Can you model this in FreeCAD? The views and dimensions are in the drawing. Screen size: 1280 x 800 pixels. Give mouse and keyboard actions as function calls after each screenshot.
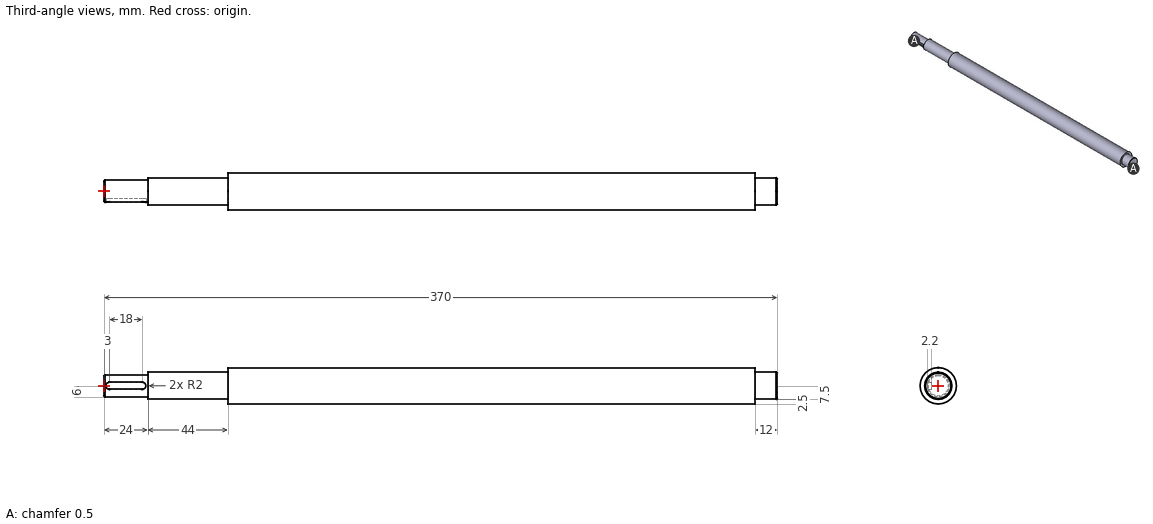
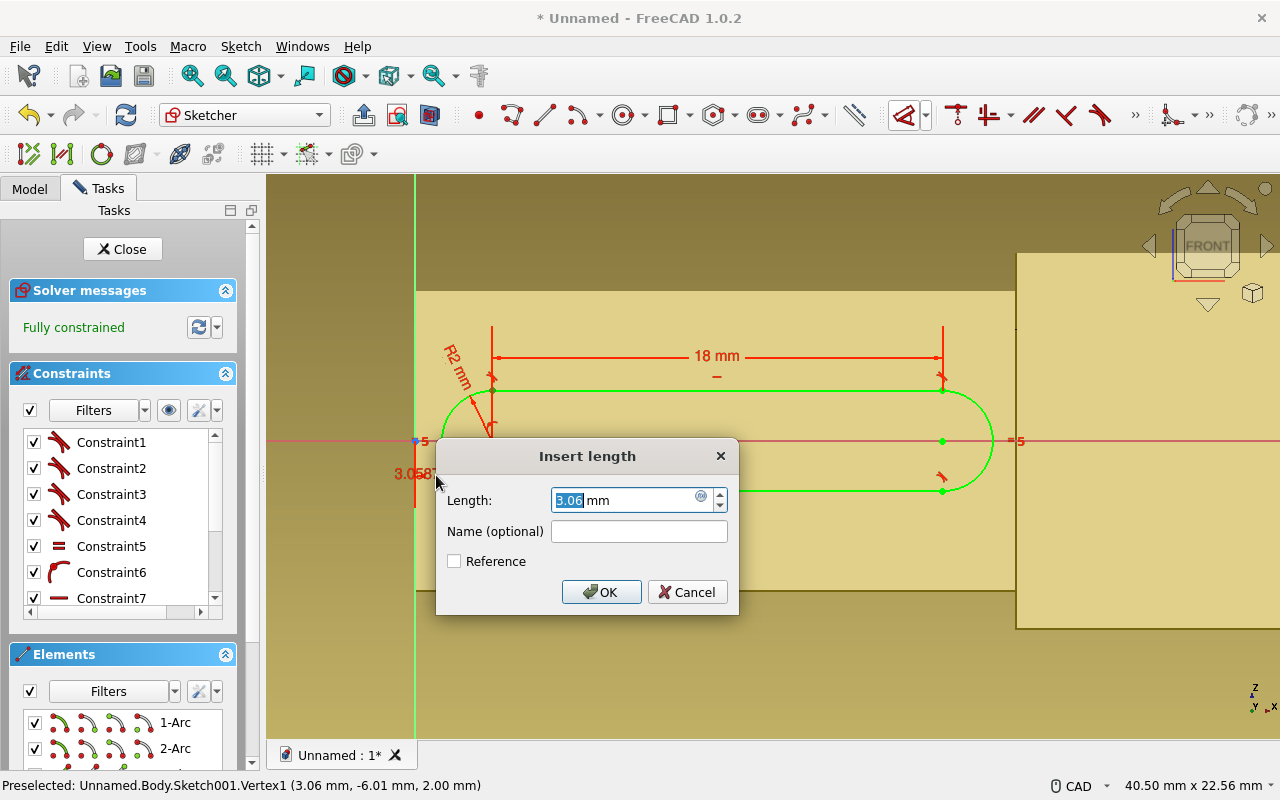
text(3)
key(Return)
key(Escape)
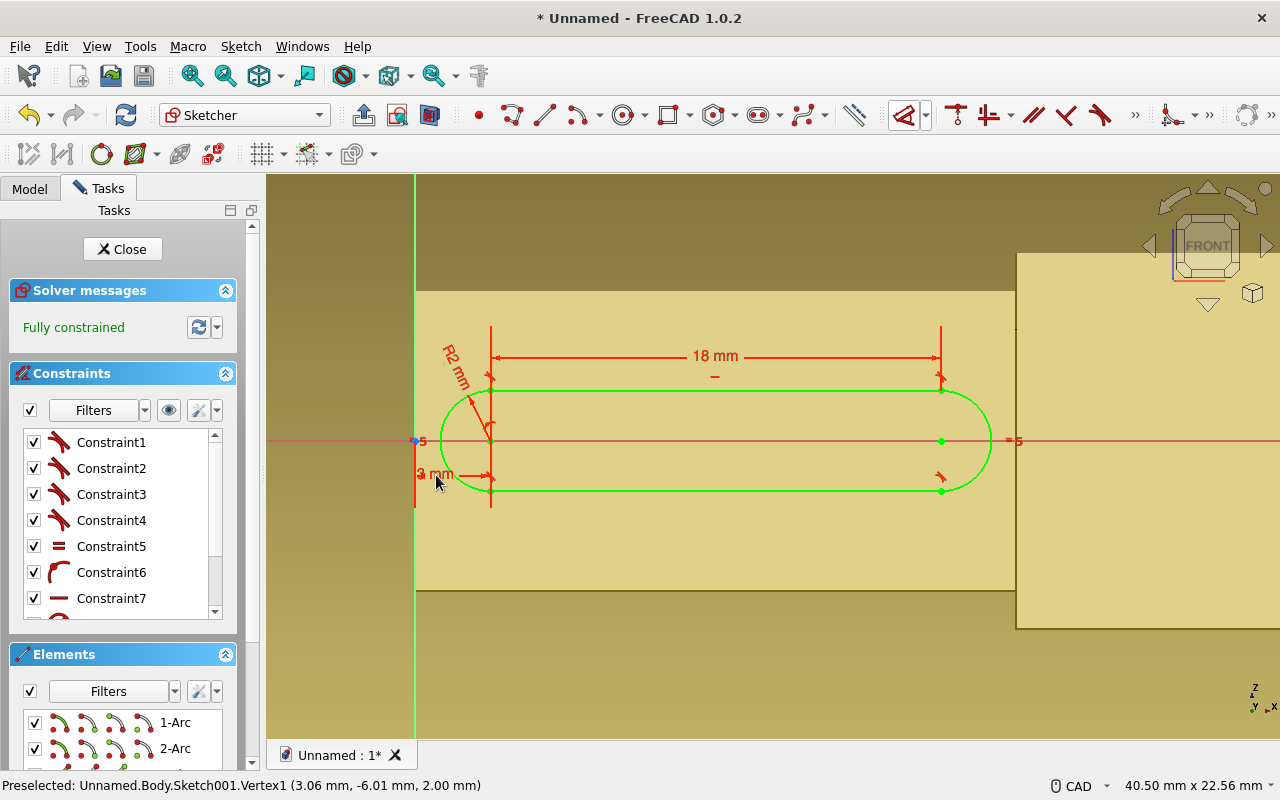
click(123, 249)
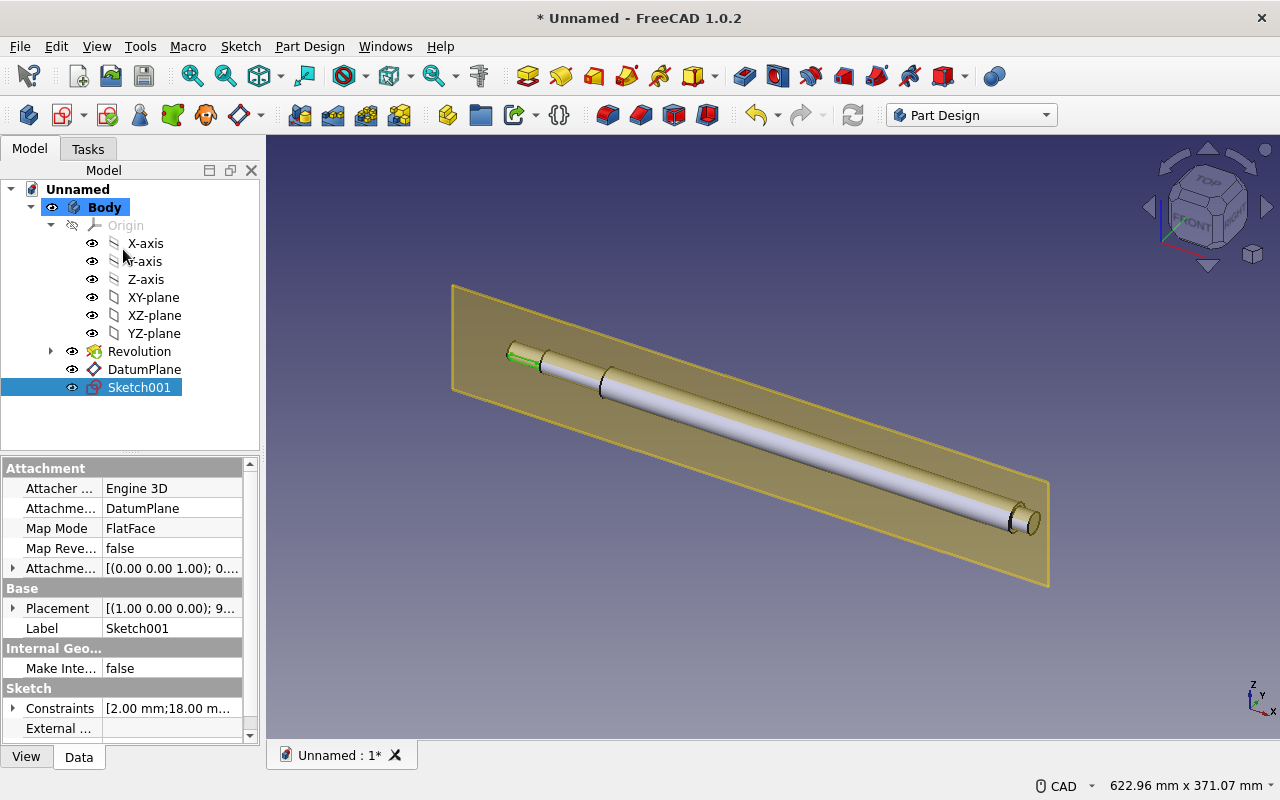
click(745, 76)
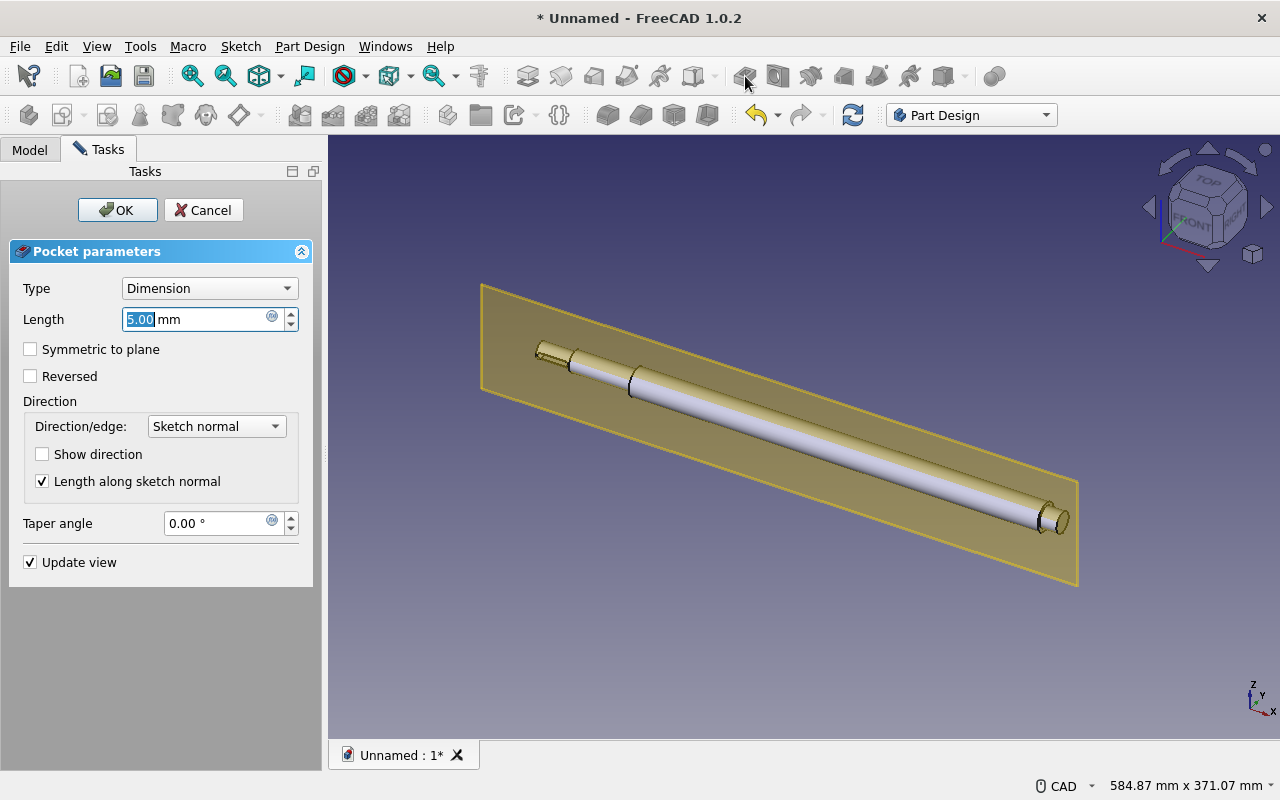
text(2.2)
key(Tab)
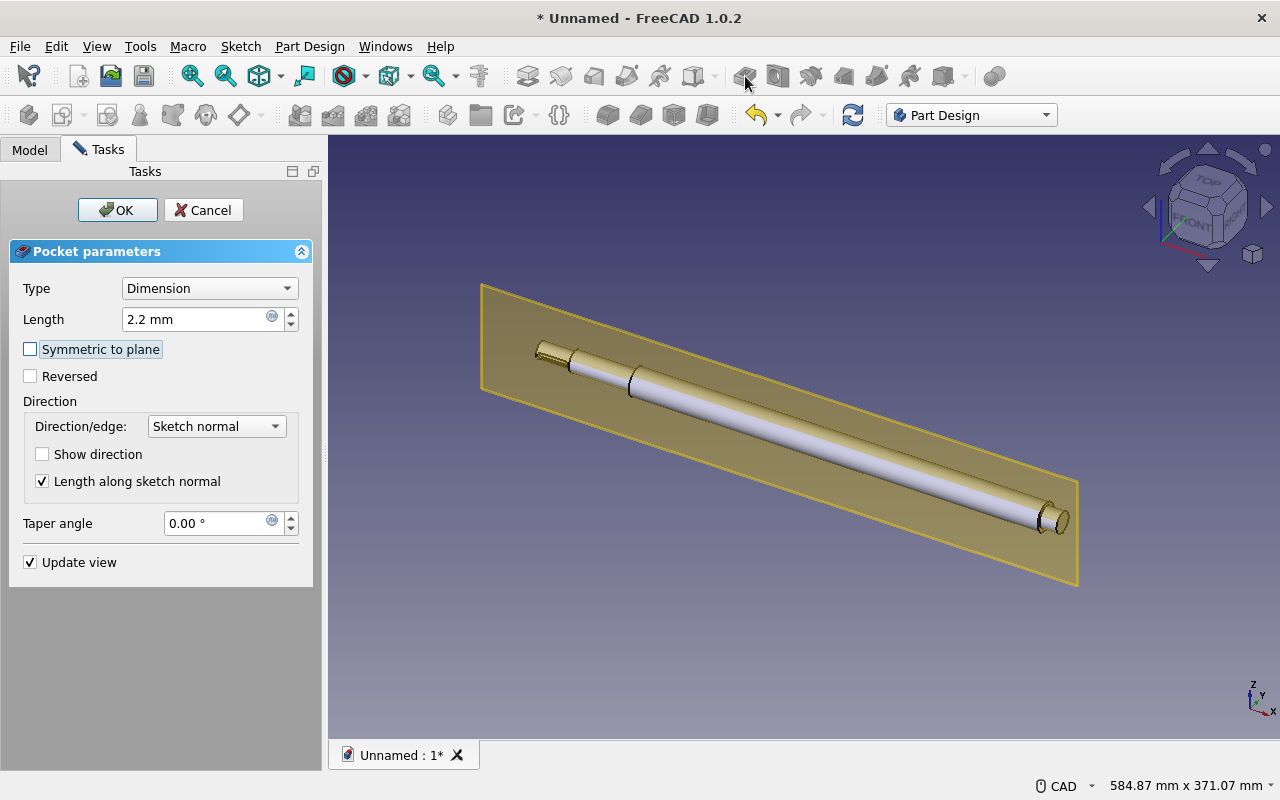
click(118, 210)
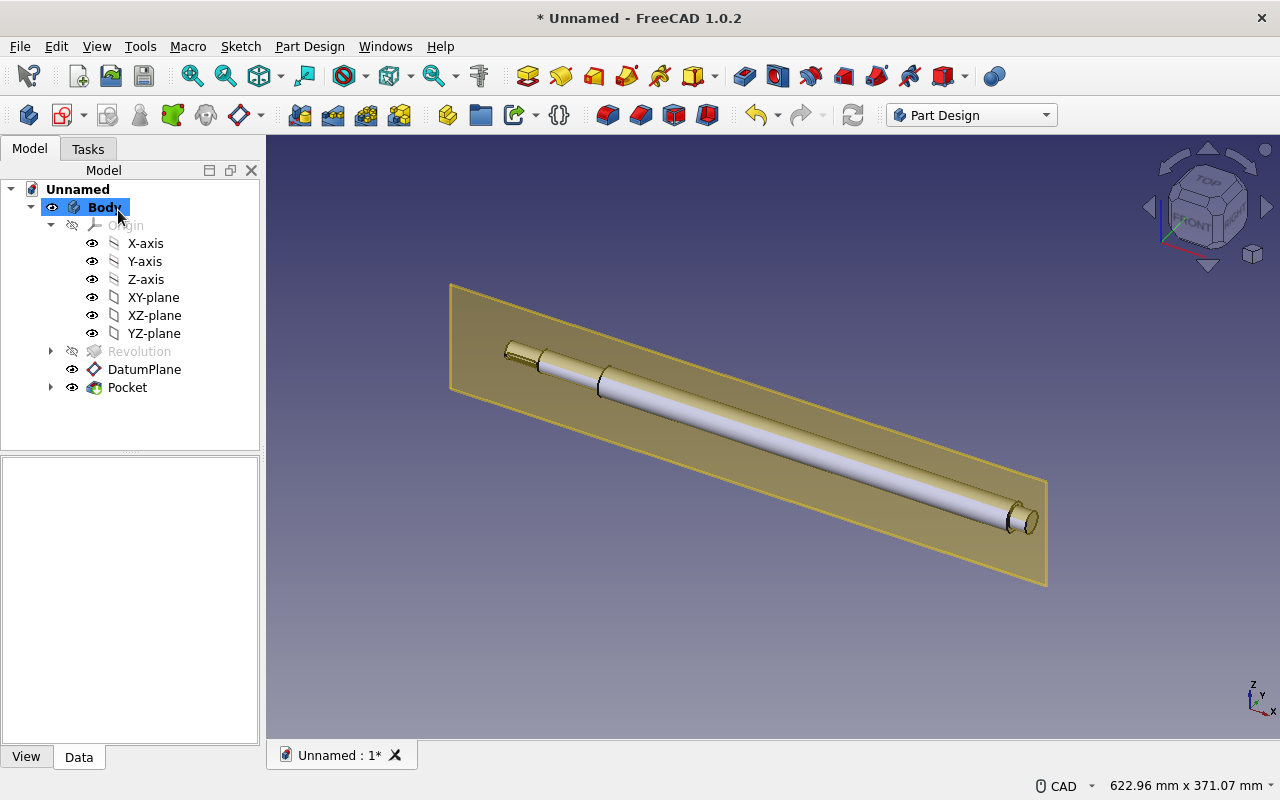
click(117, 369)
key(space)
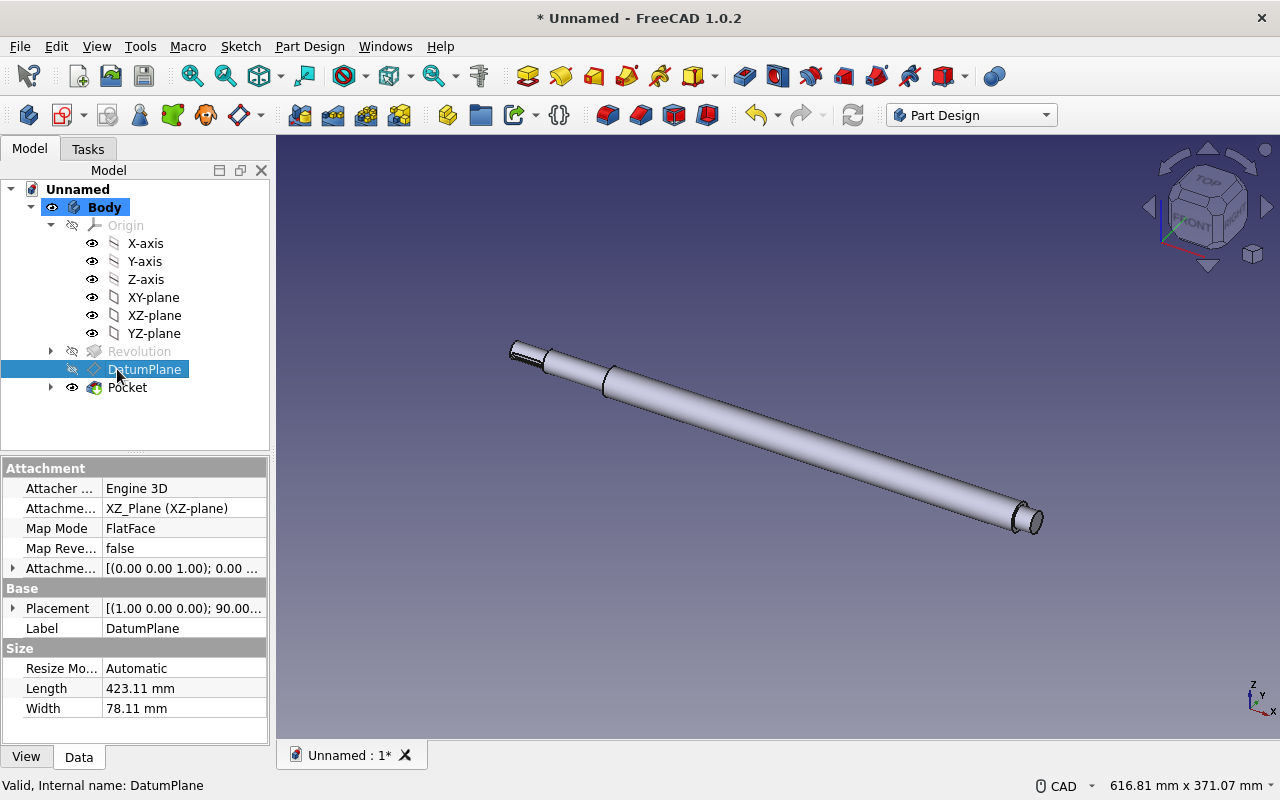
click(515, 341)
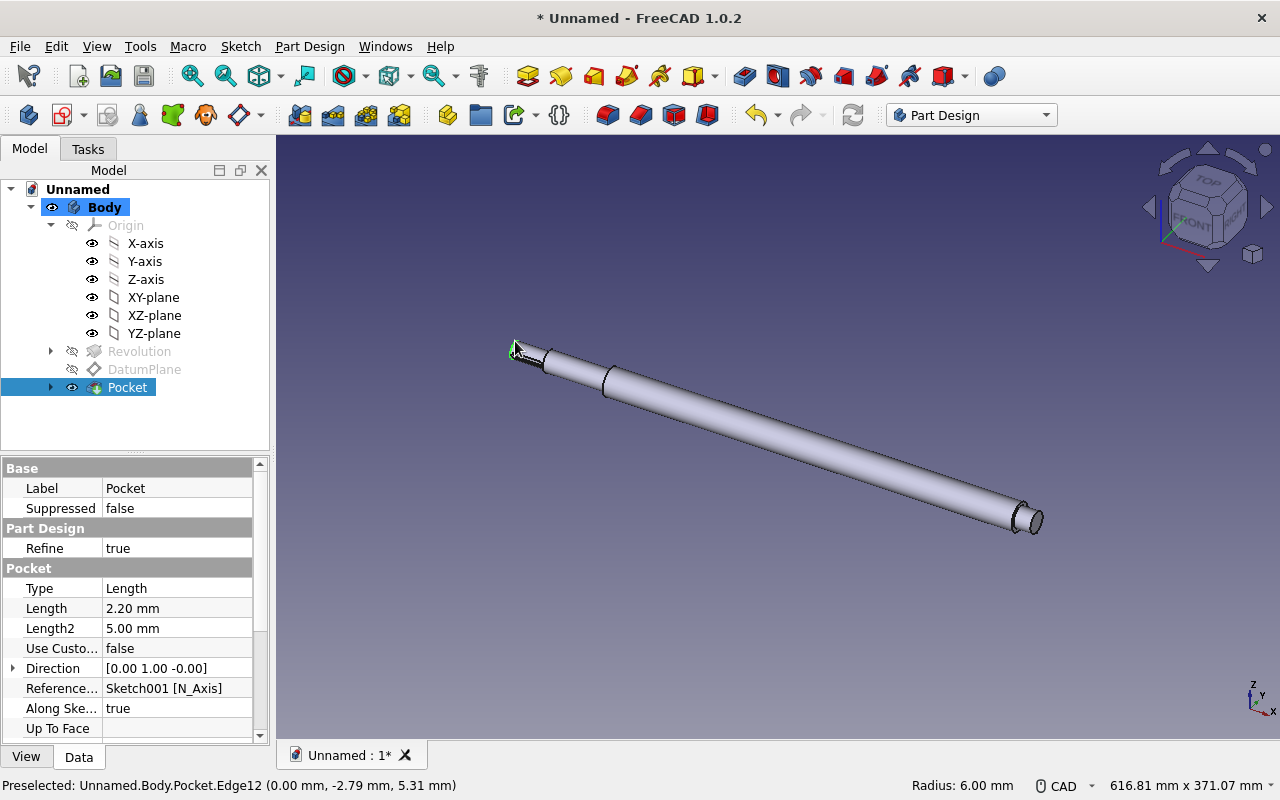
click(1037, 512, ctrl)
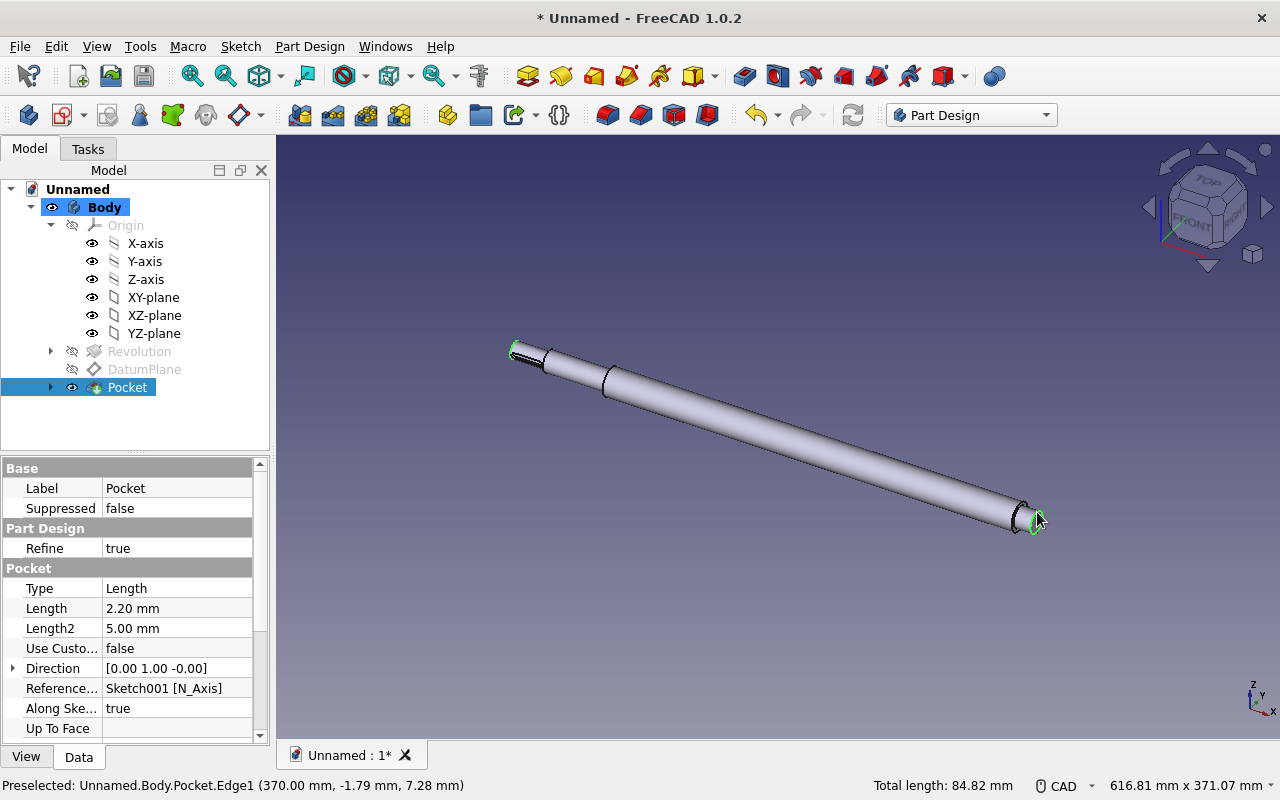
click(641, 116)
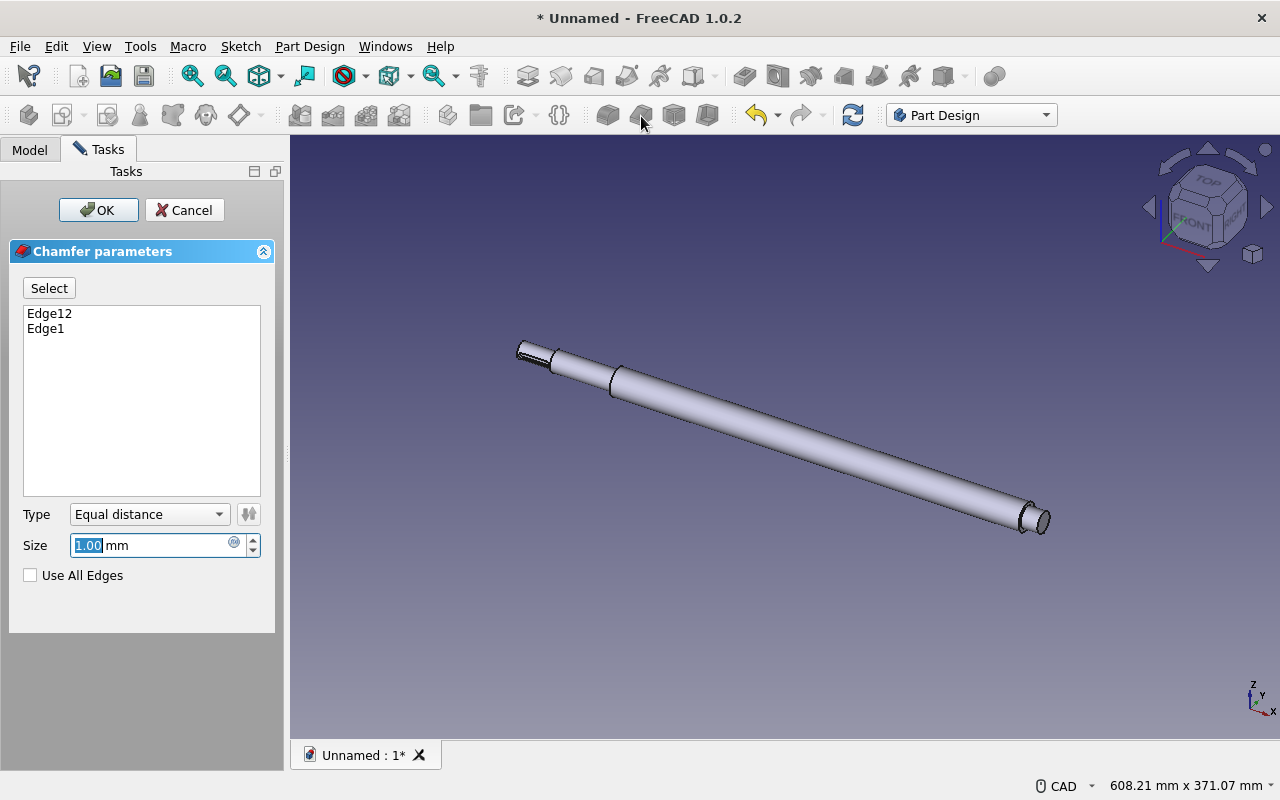
text(0.5)
key(Tab)